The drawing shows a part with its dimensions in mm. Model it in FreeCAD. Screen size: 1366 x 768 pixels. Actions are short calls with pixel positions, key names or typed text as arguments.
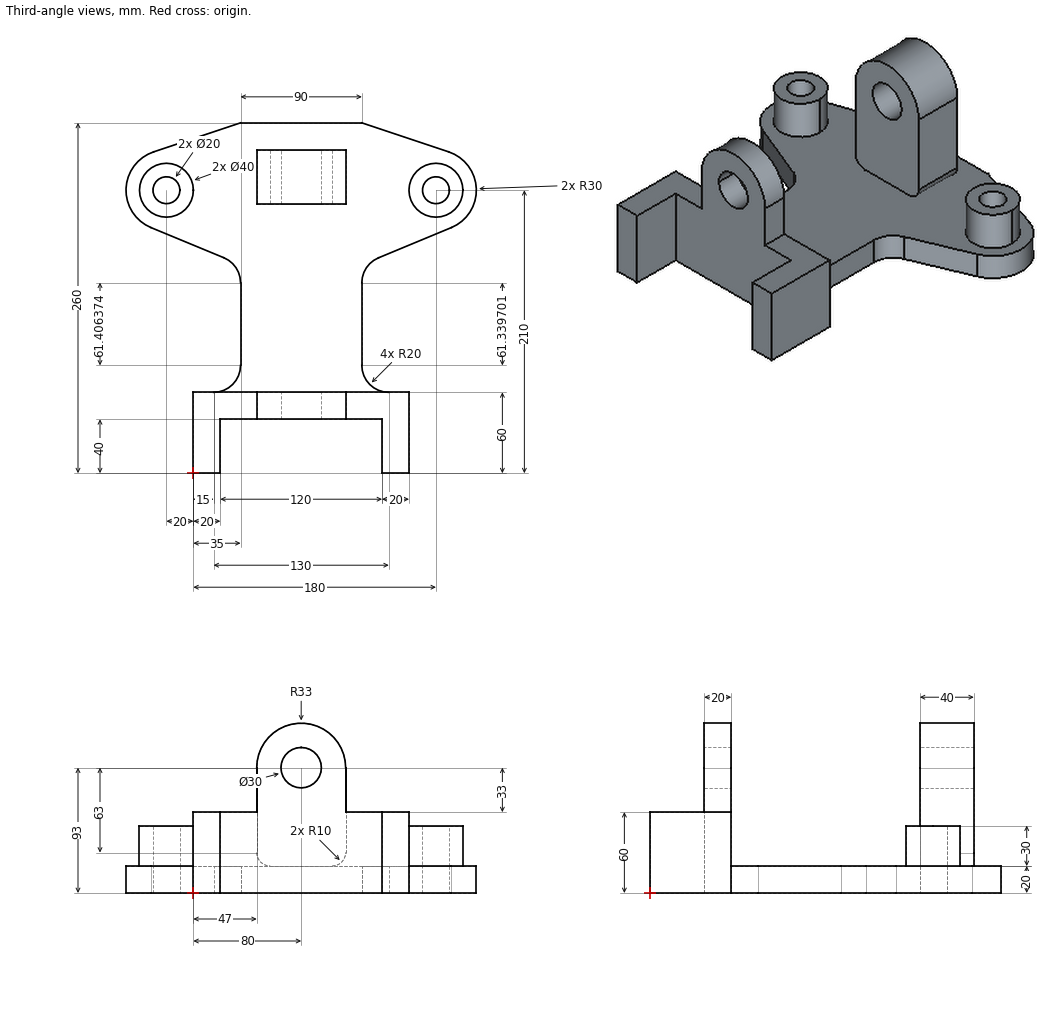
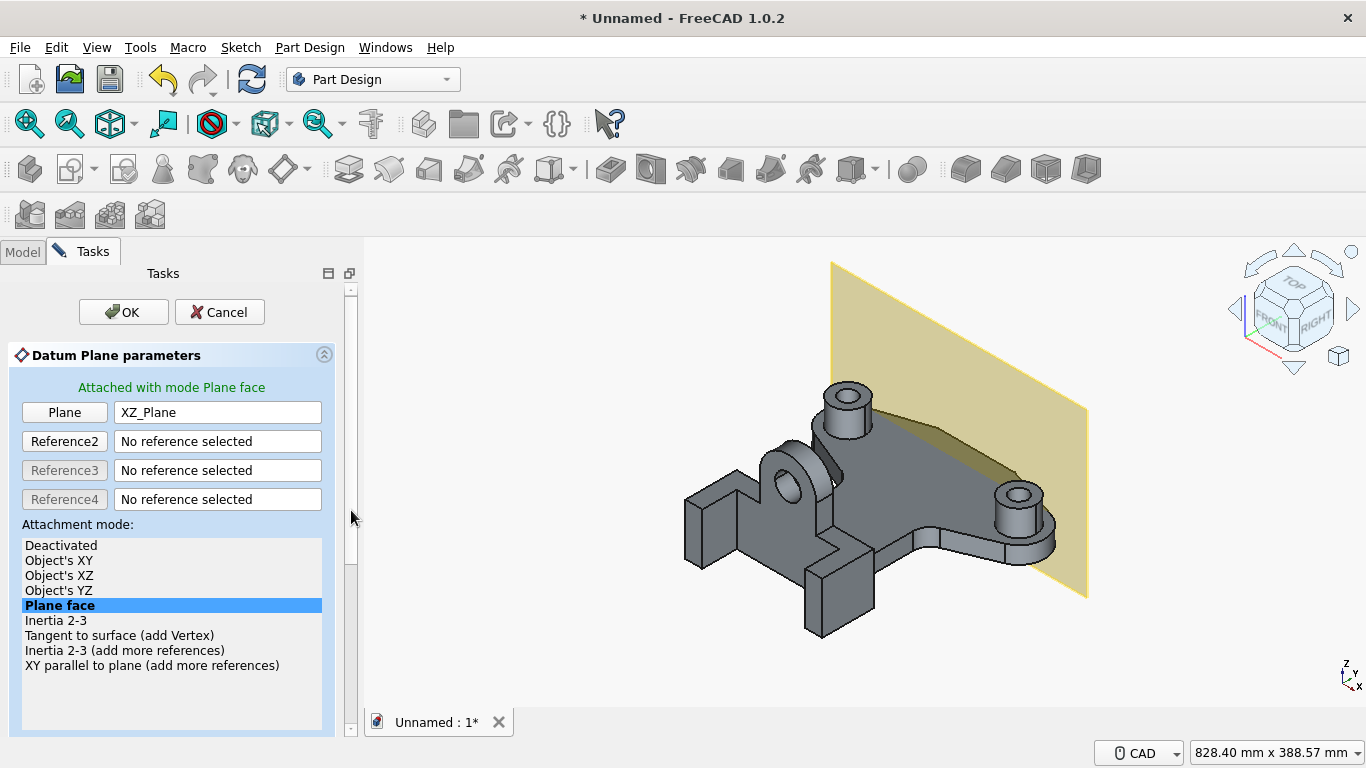
click(124, 312)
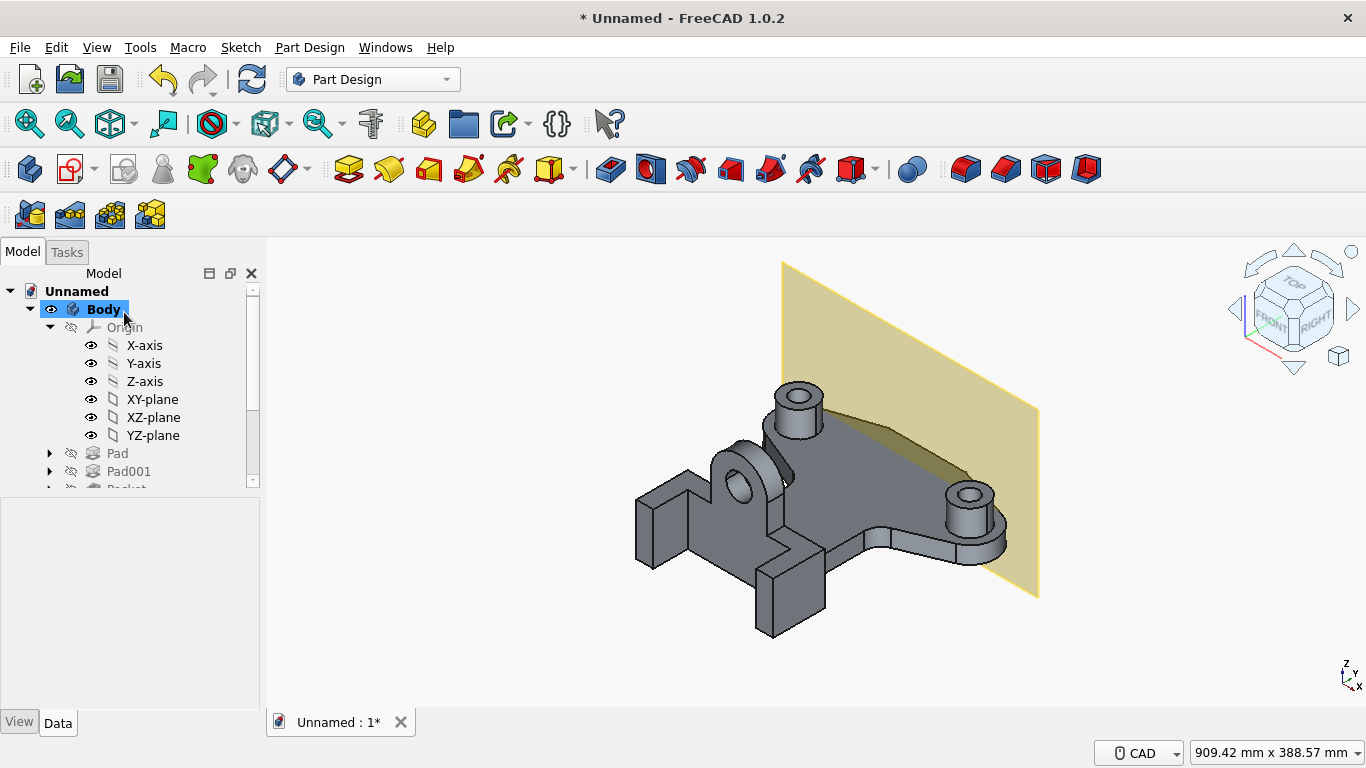
scroll(100, 377, down, 3)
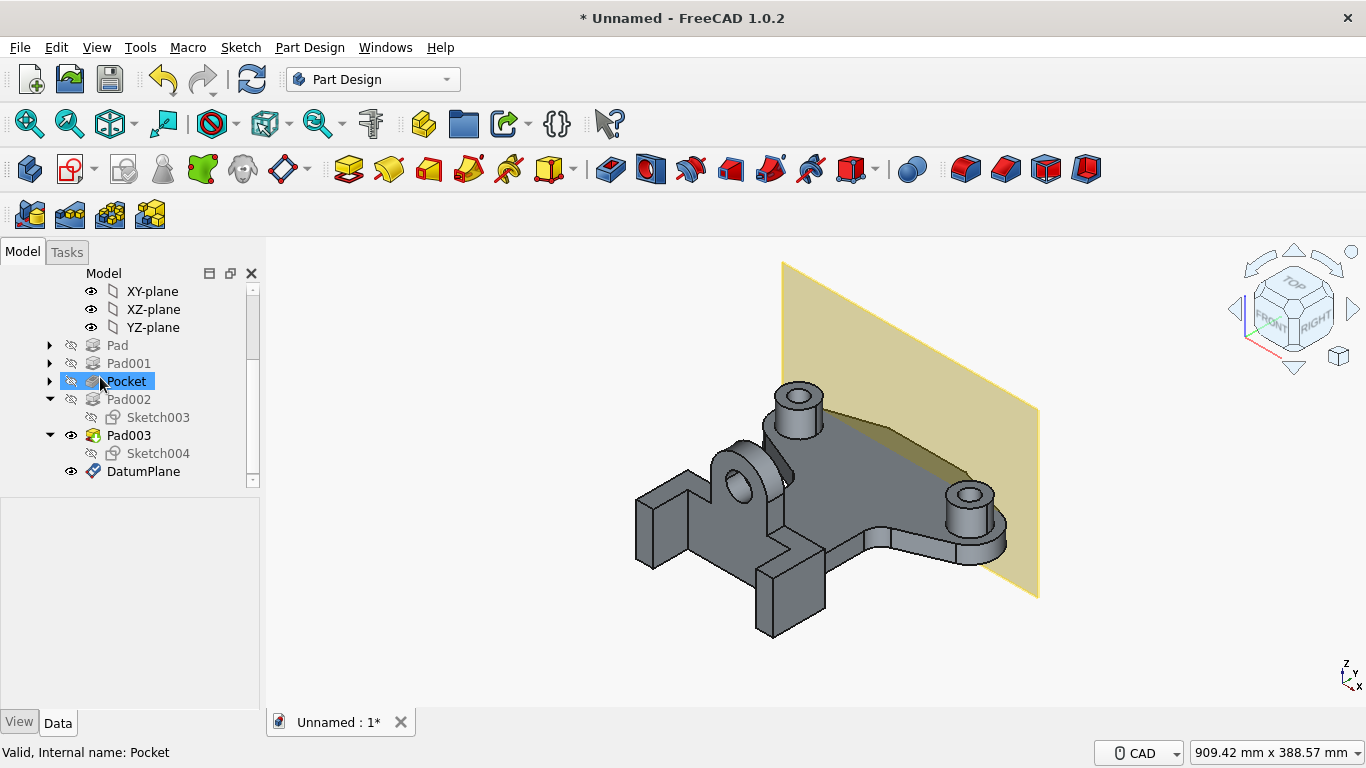
click(116, 471)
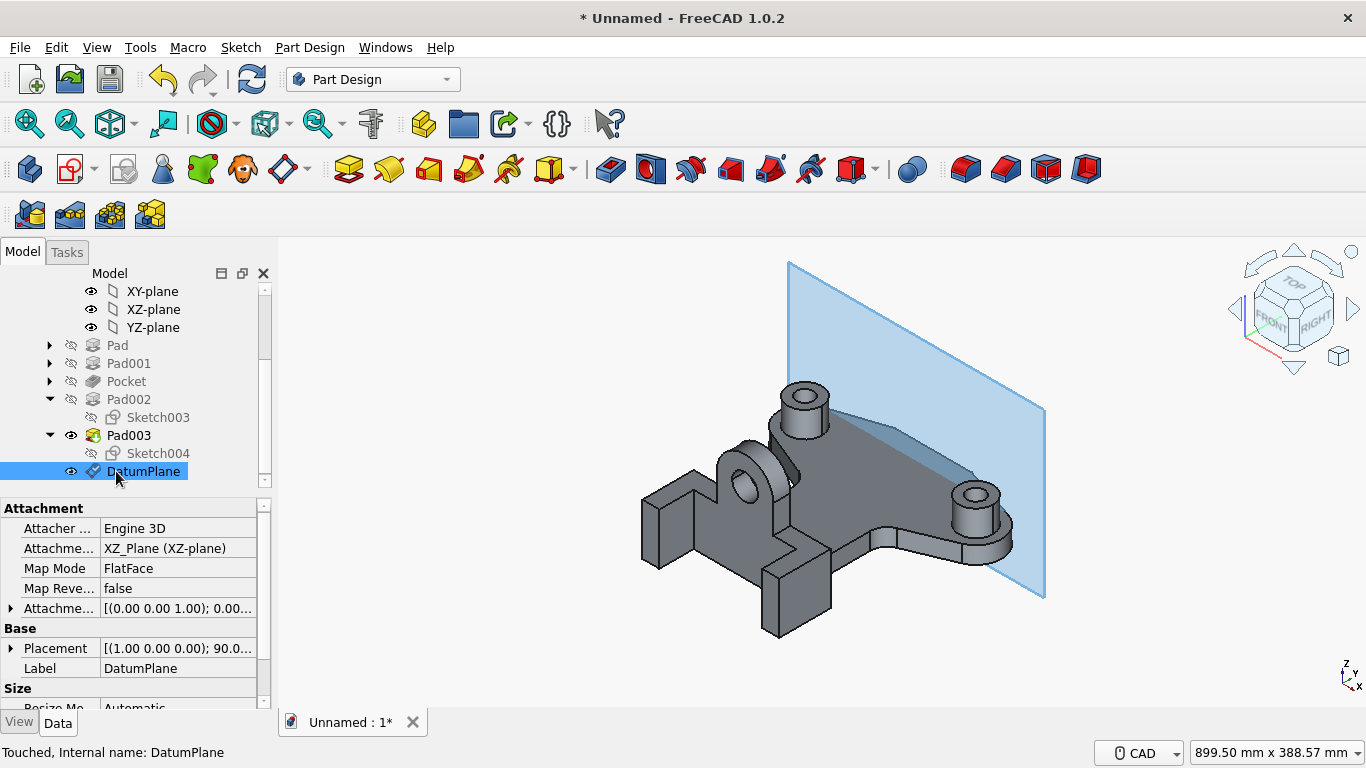
click(70, 170)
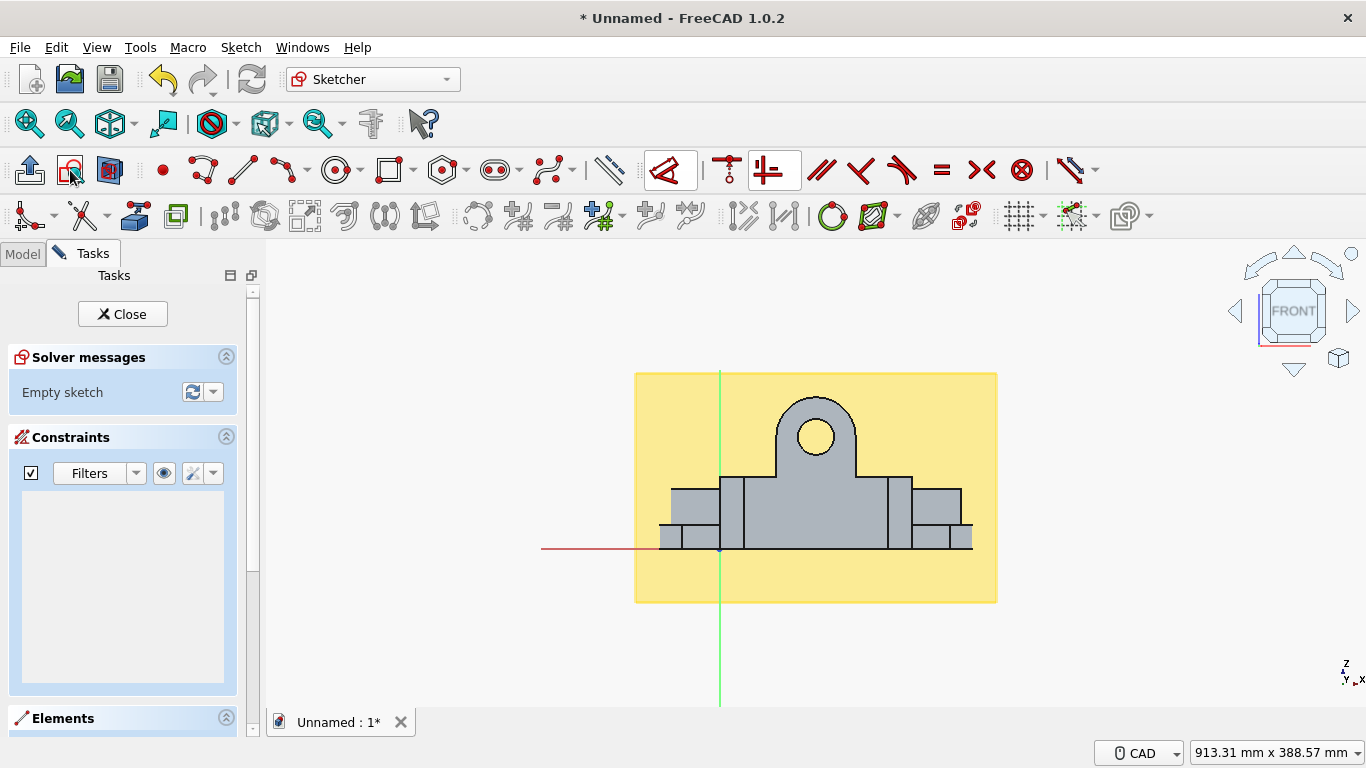
click(110, 170)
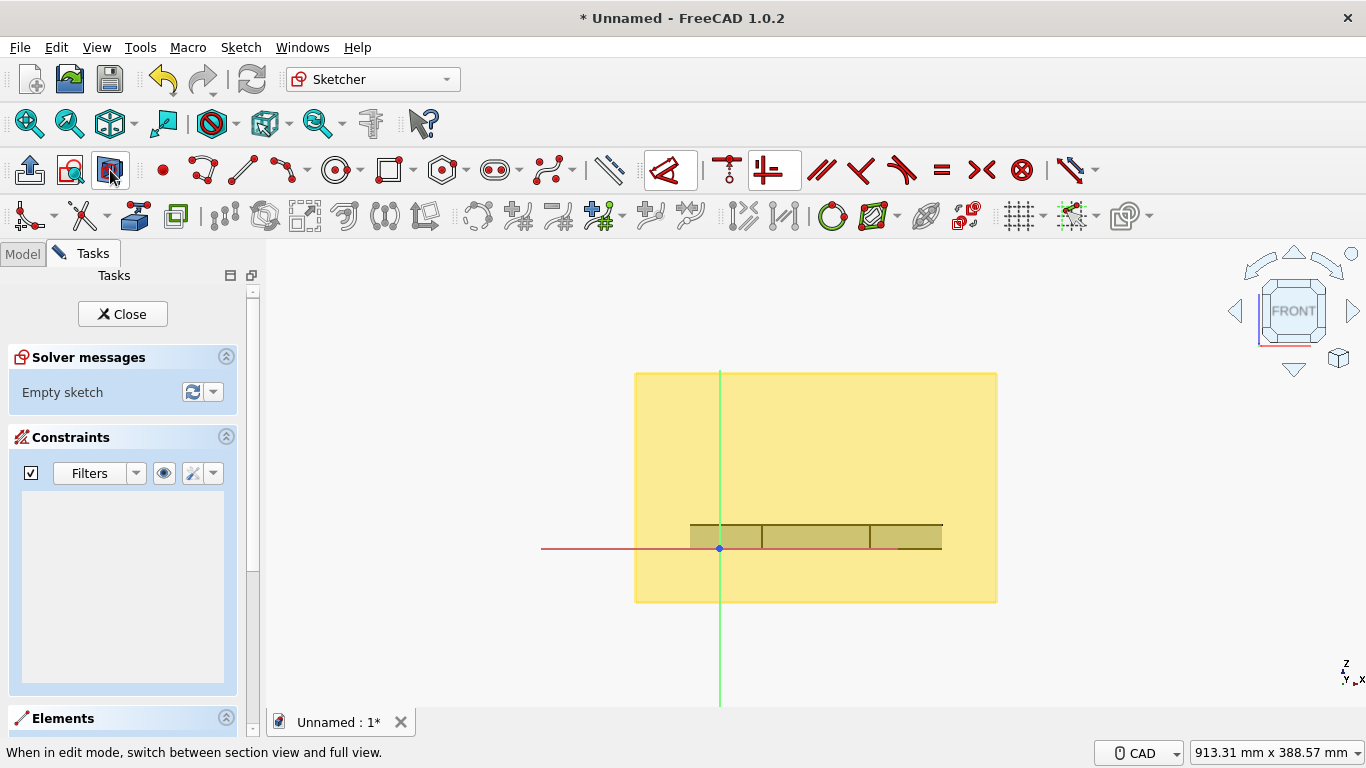
scroll(837, 473, up, 3)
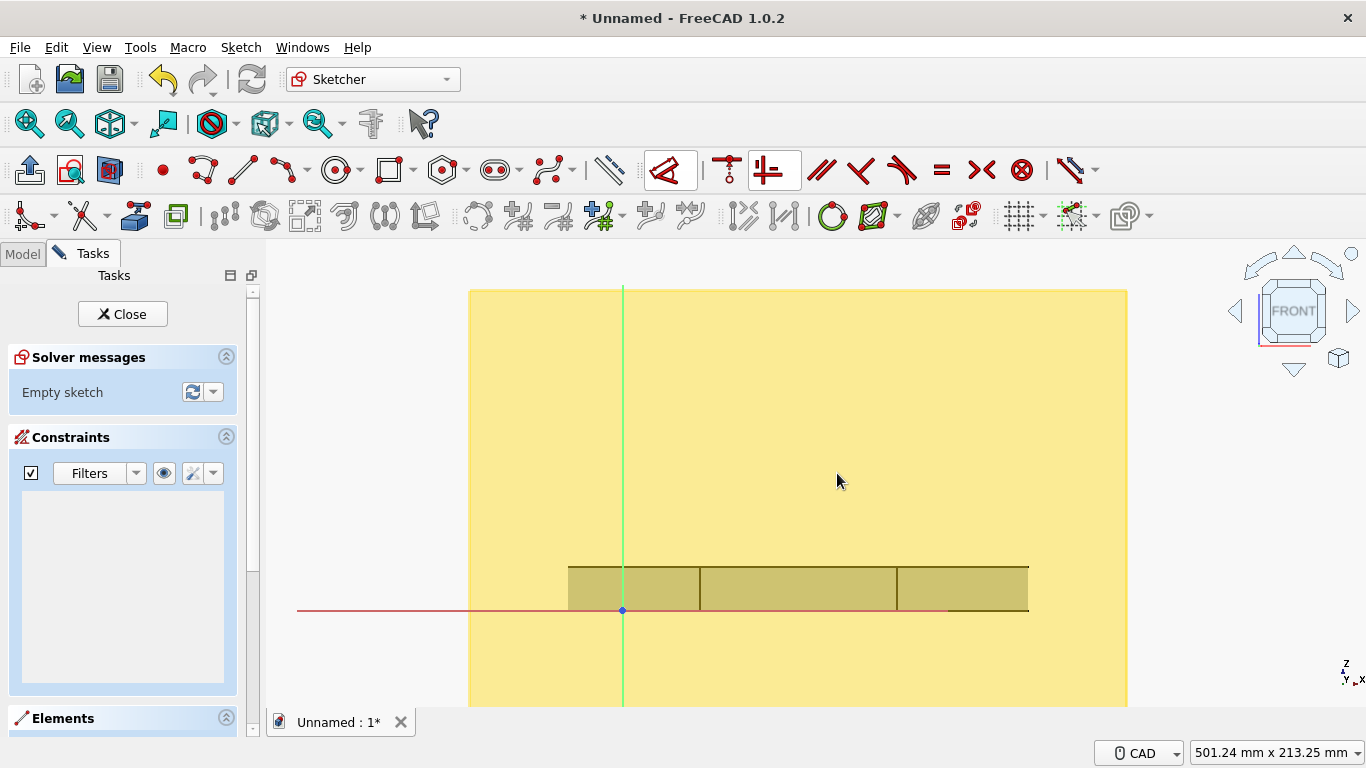
click(244, 170)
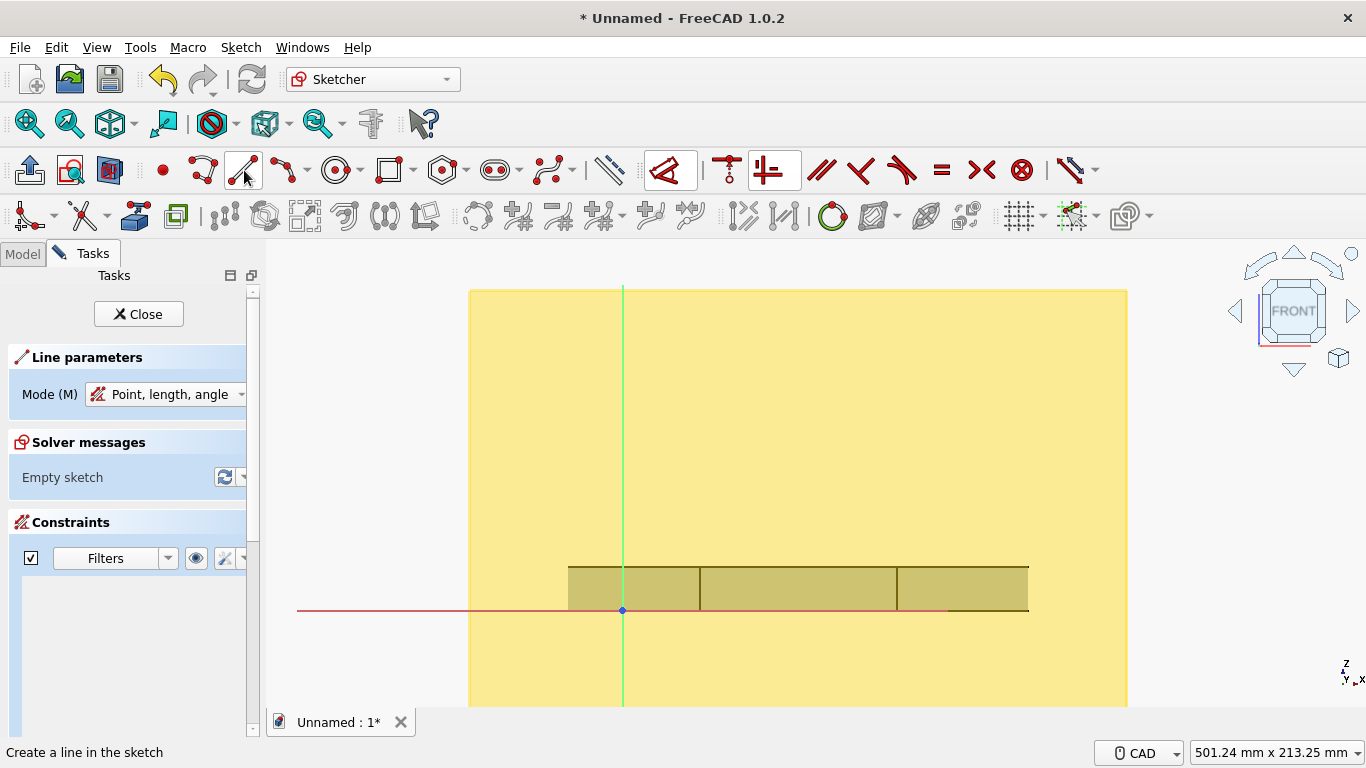
click(726, 545)
click(726, 407)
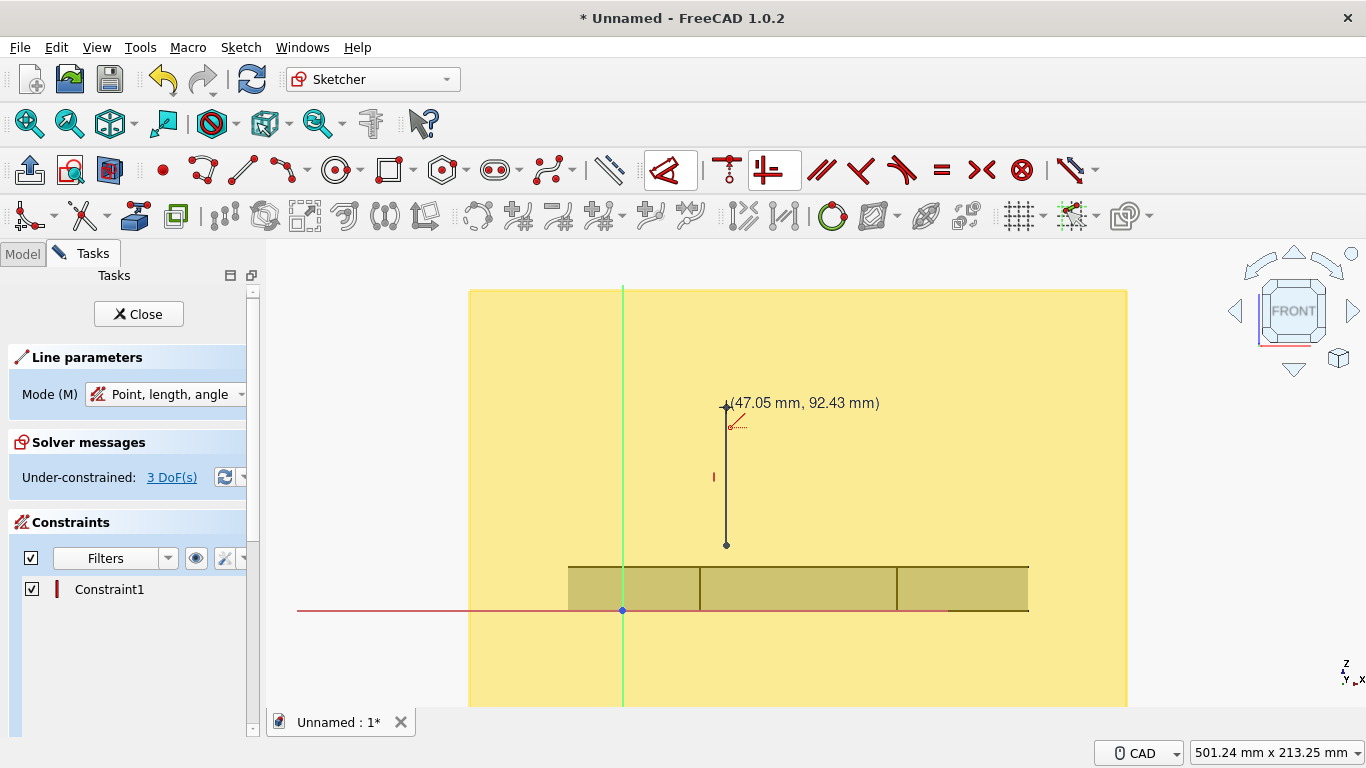
click(871, 407)
click(871, 545)